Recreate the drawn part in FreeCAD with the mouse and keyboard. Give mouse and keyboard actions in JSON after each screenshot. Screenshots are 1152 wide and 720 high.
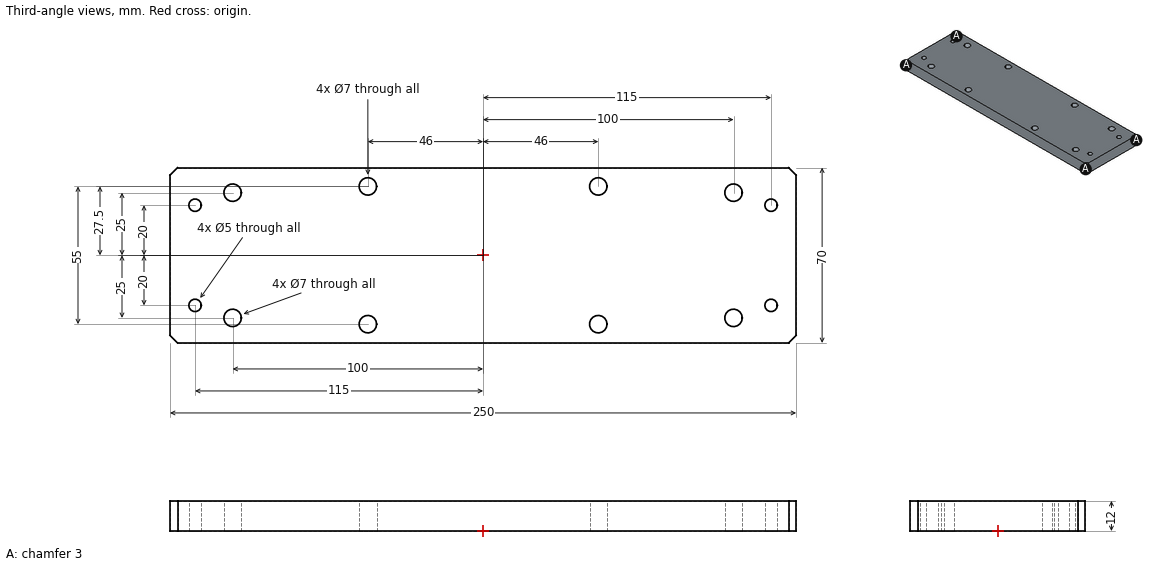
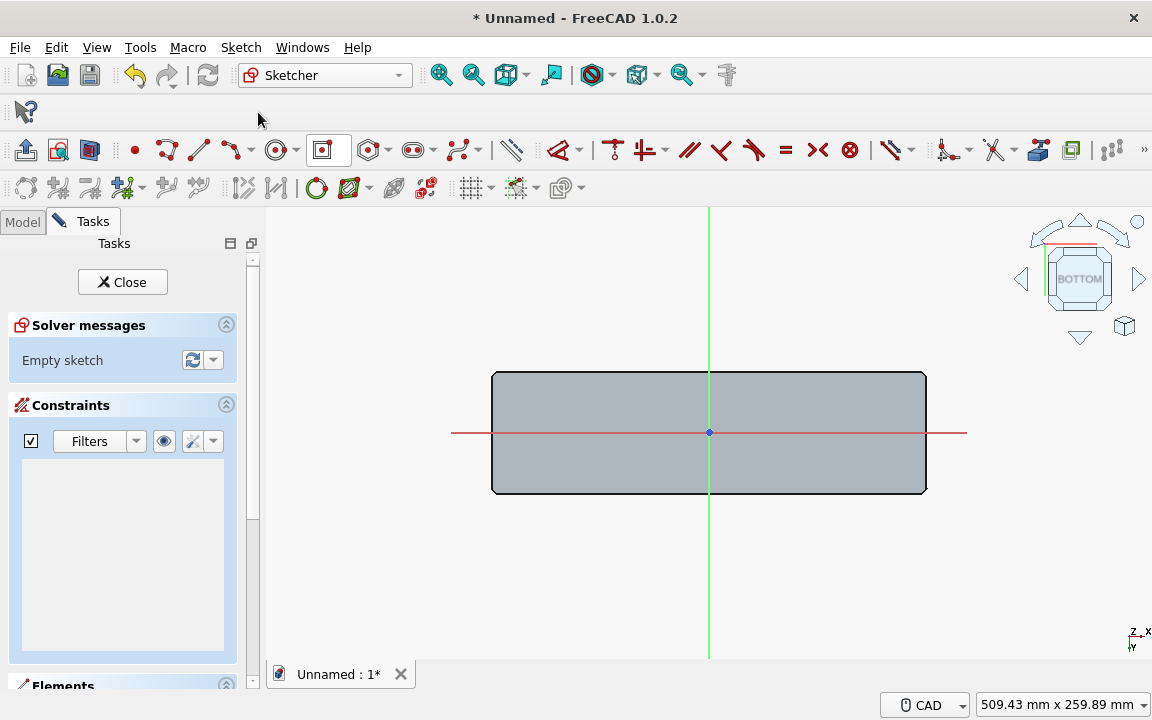
{"action": "scroll", "coordinate": [848, 433], "scroll_direction": "up", "scroll_amount": 2}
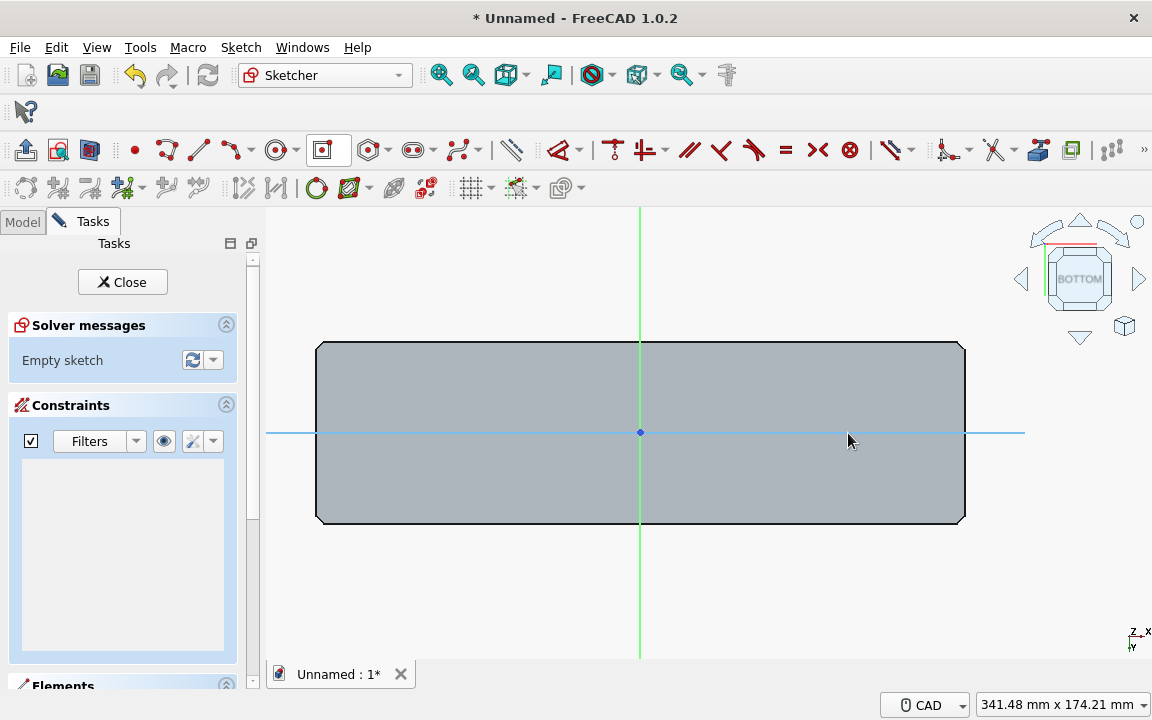
{"action": "left_click", "coordinate": [276, 150]}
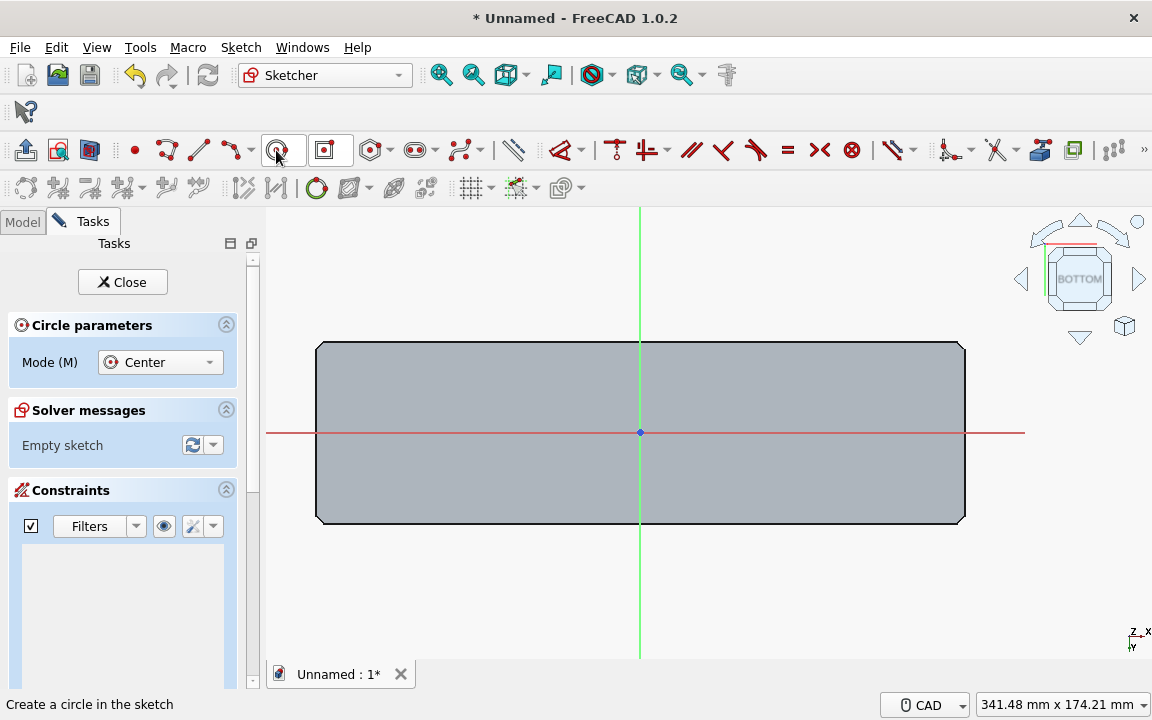
{"action": "scroll", "coordinate": [381, 368], "scroll_direction": "up", "scroll_amount": 5}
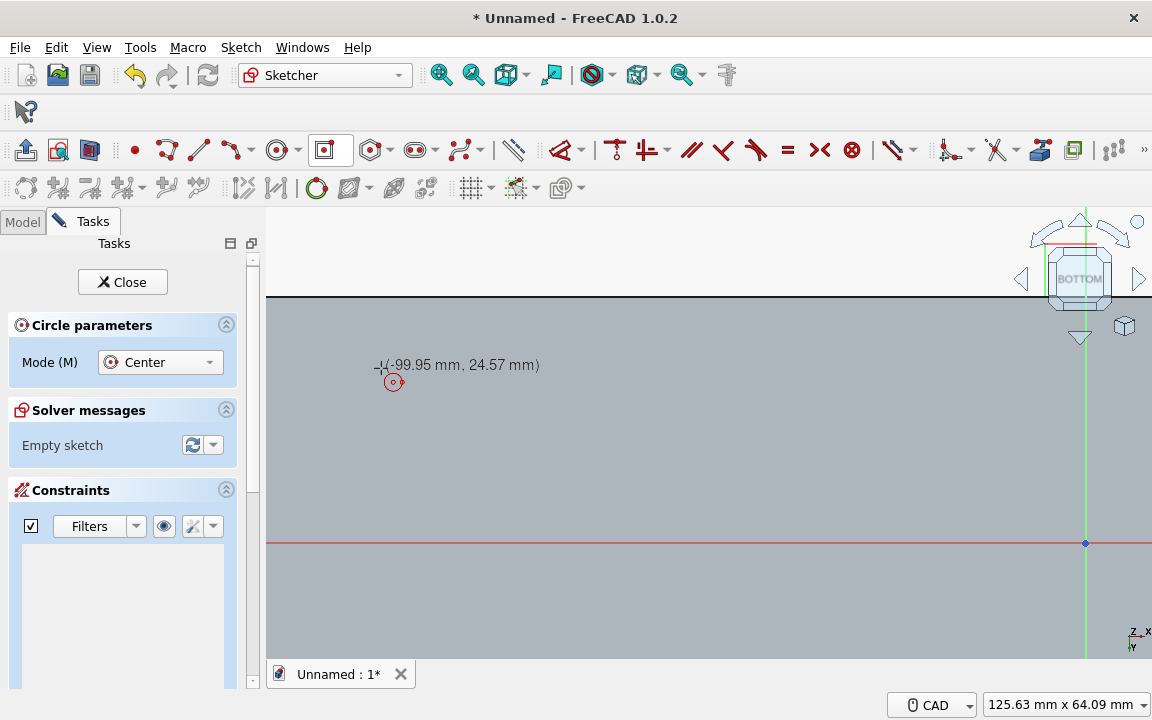
{"action": "left_click", "coordinate": [380, 367]}
{"action": "left_click", "coordinate": [398, 350]}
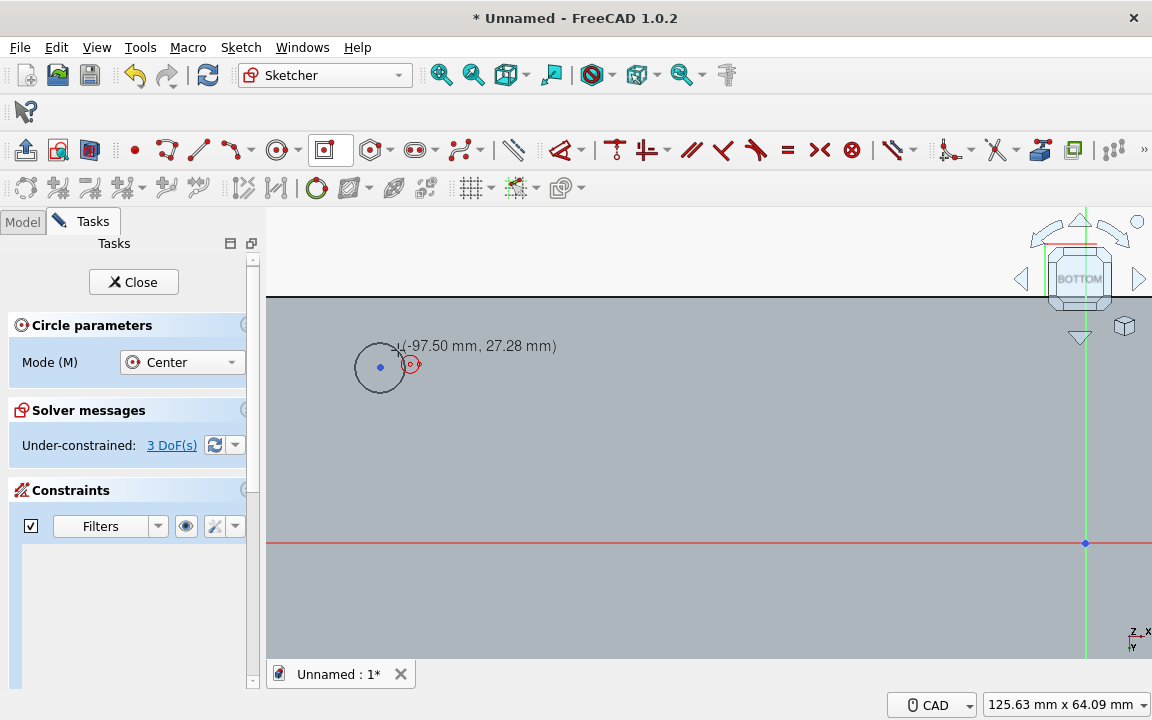
{"action": "scroll", "coordinate": [381, 369], "scroll_direction": "down", "scroll_amount": 5}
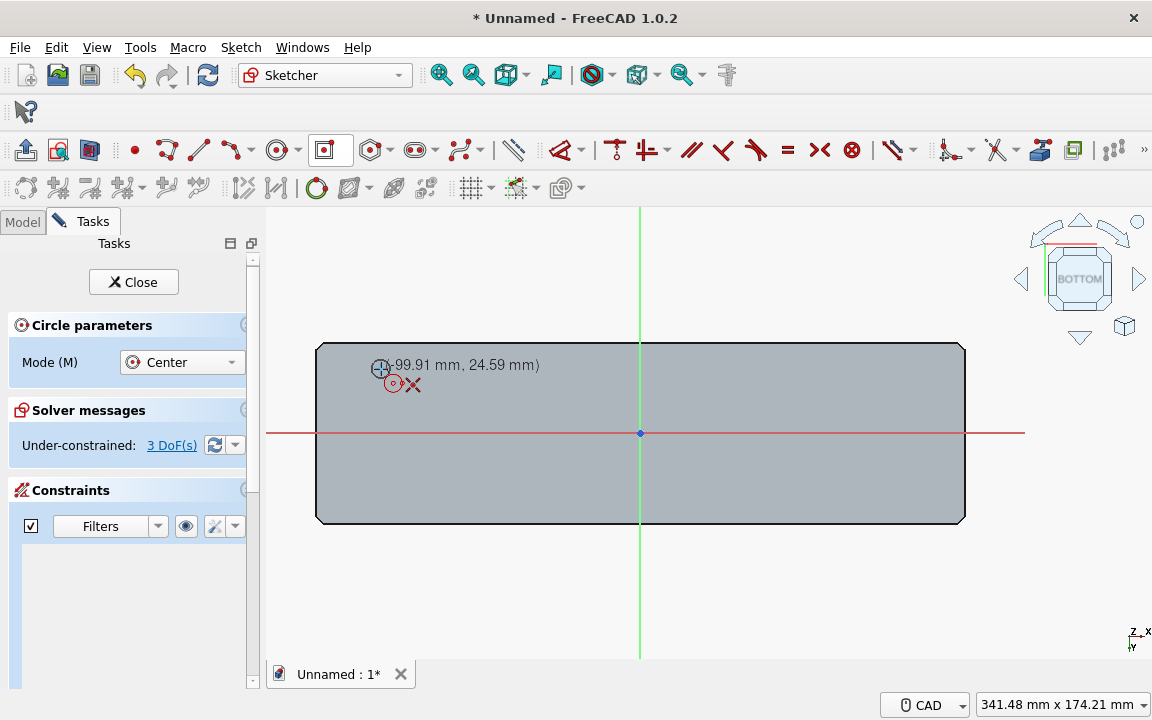
{"action": "scroll", "coordinate": [381, 498], "scroll_direction": "up", "scroll_amount": 5}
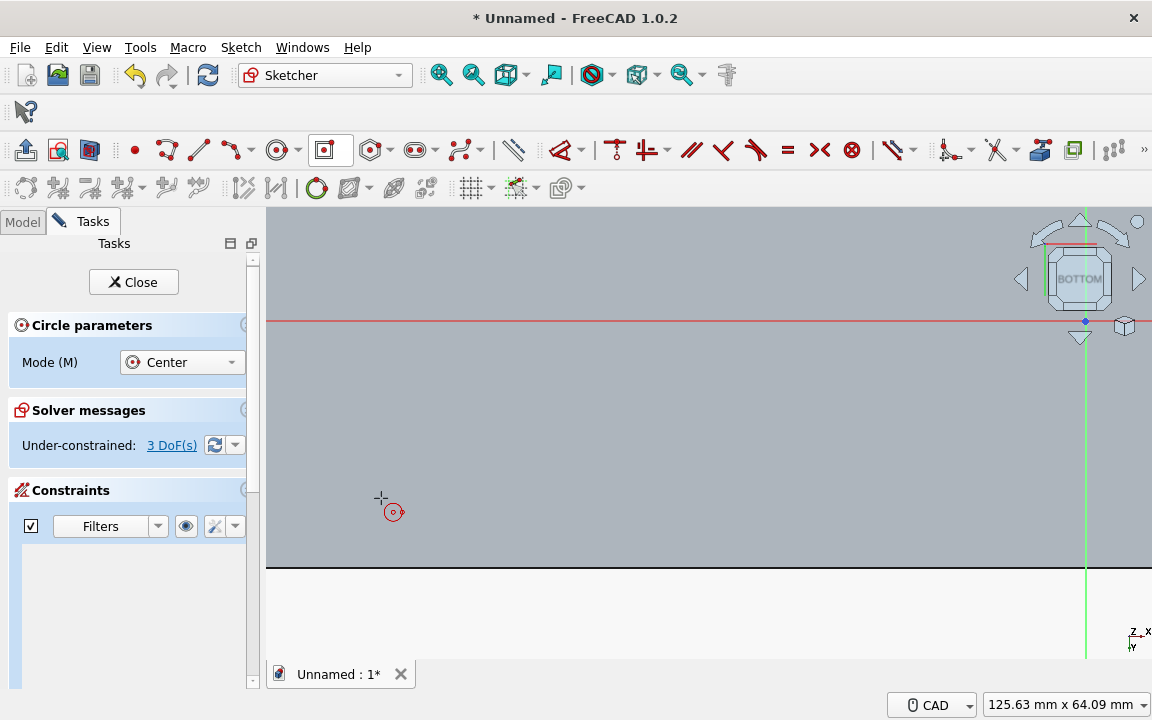
{"action": "left_click", "coordinate": [380, 498]}
{"action": "left_click", "coordinate": [398, 480]}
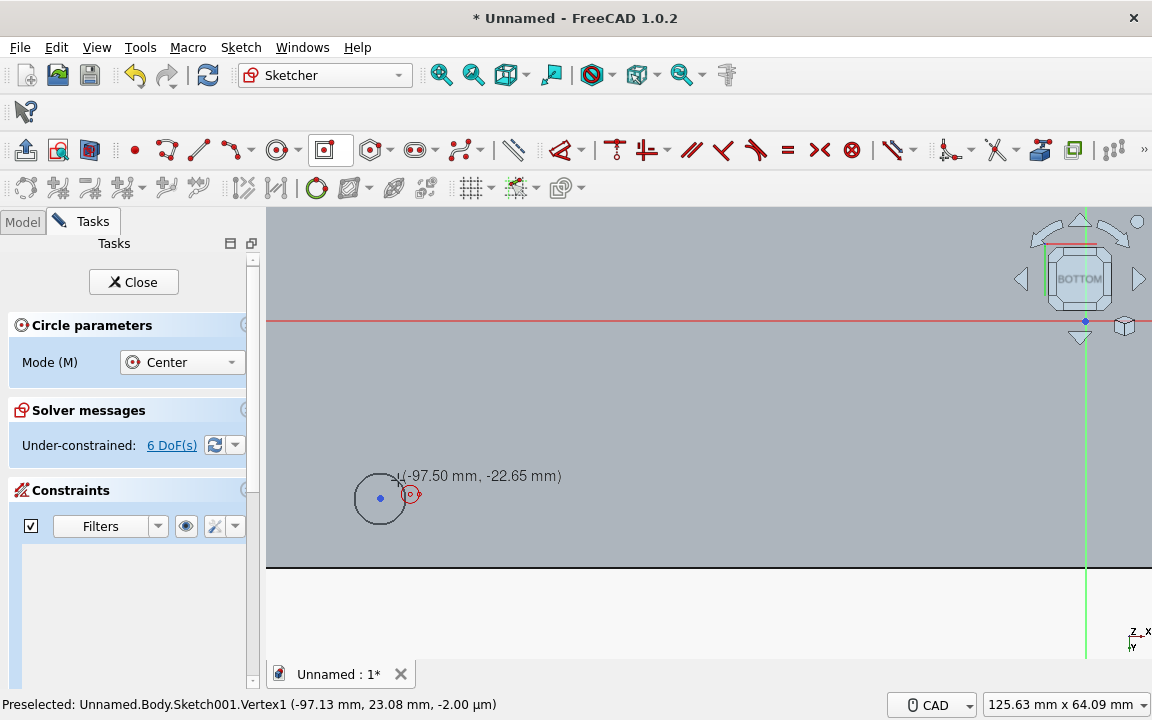
{"action": "scroll", "coordinate": [381, 498], "scroll_direction": "down", "scroll_amount": 5}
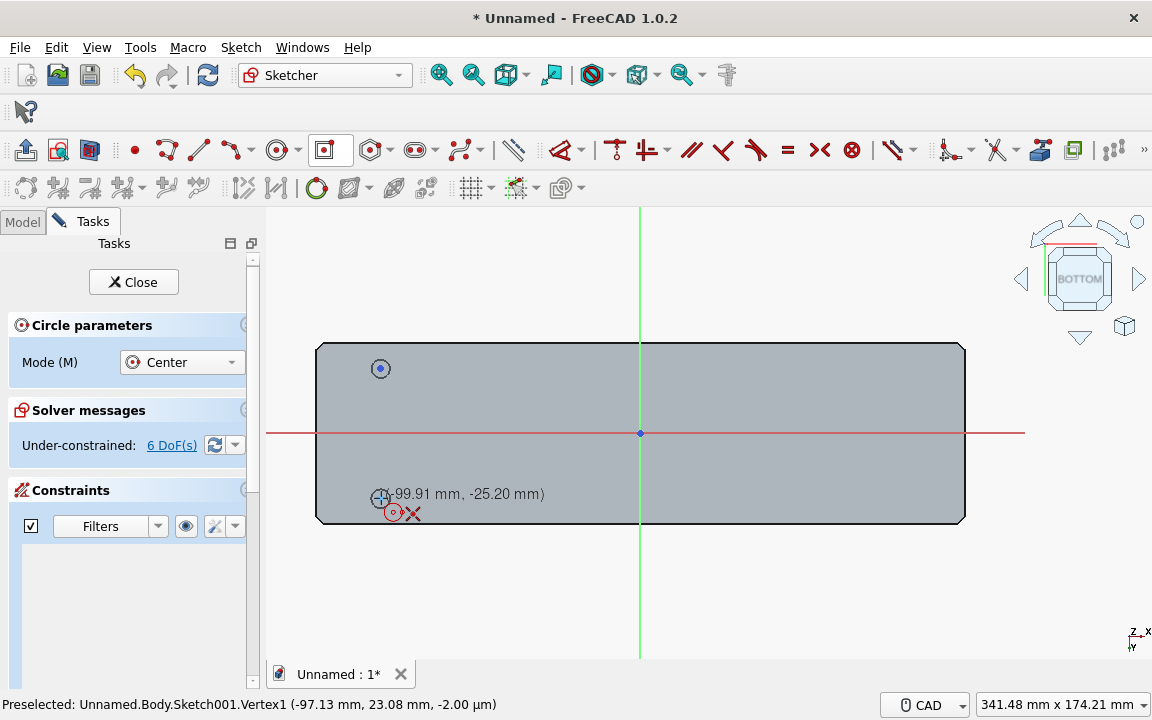
{"action": "scroll", "coordinate": [900, 498], "scroll_direction": "up", "scroll_amount": 5}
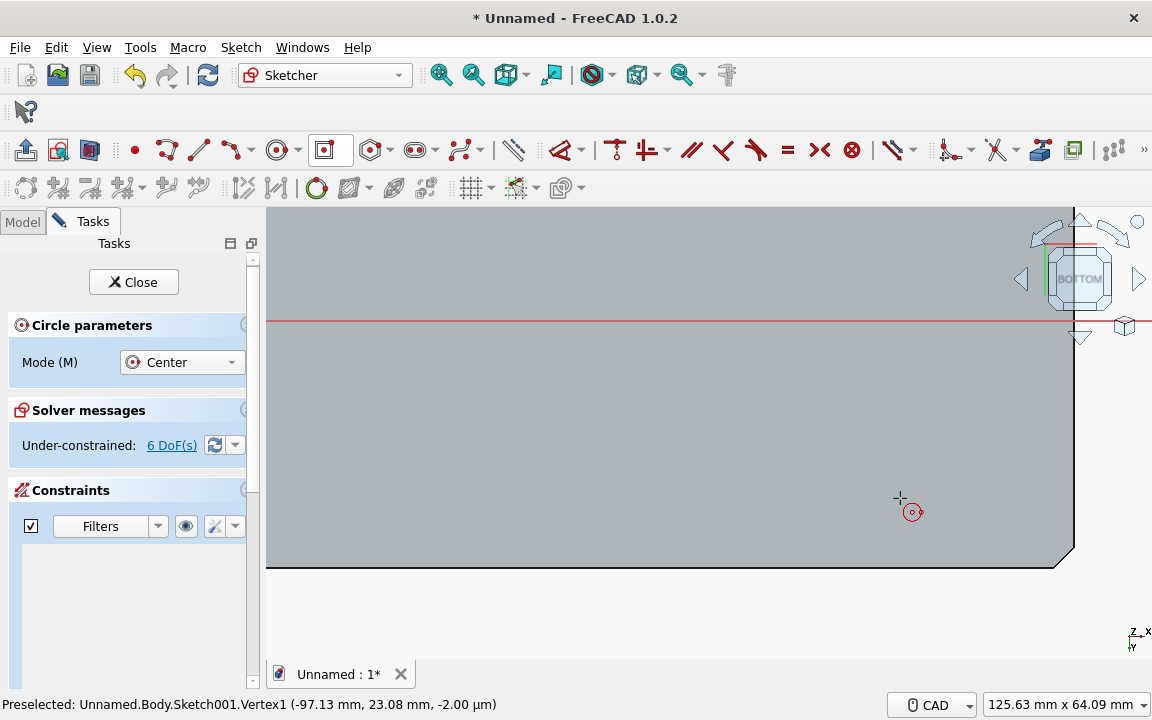
{"action": "left_click", "coordinate": [898, 498]}
{"action": "left_click", "coordinate": [916, 480]}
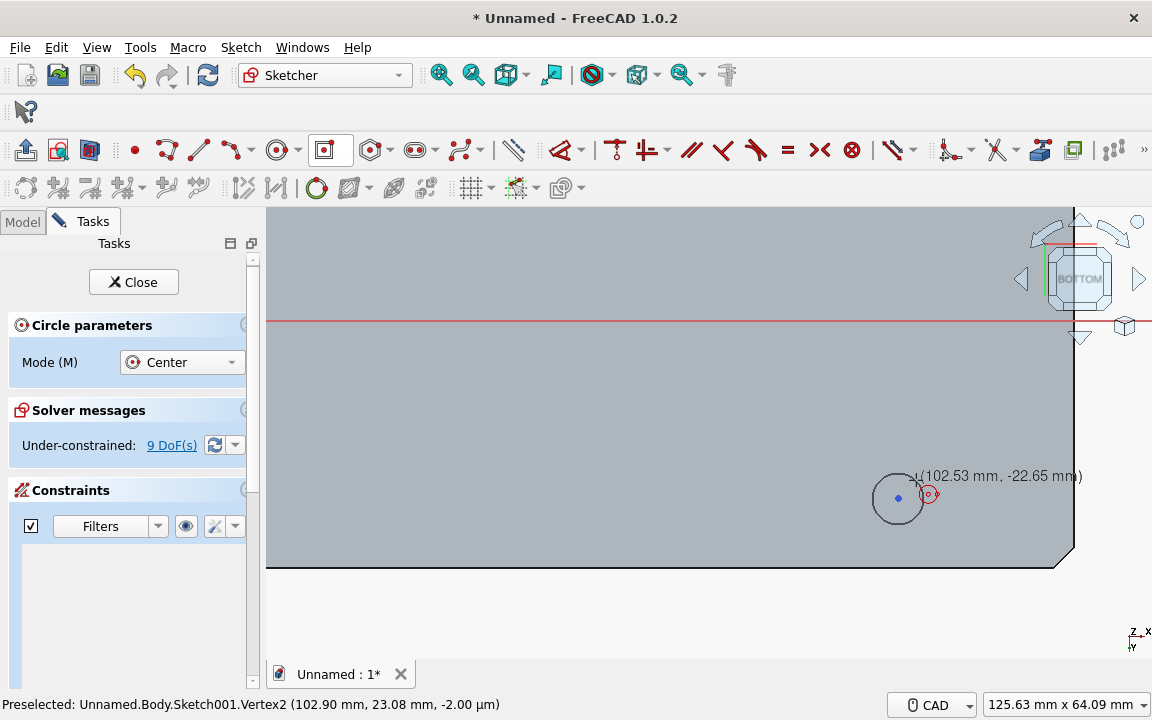
{"action": "scroll", "coordinate": [901, 498], "scroll_direction": "down", "scroll_amount": 5}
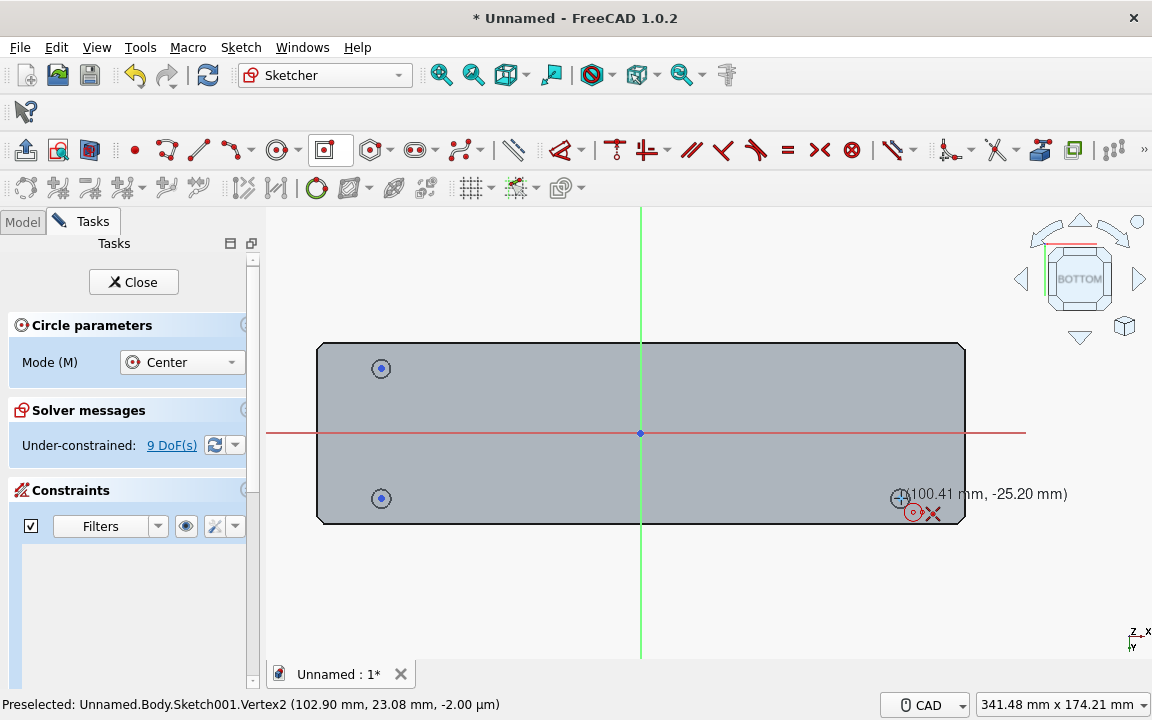
{"action": "scroll", "coordinate": [900, 369], "scroll_direction": "up", "scroll_amount": 5}